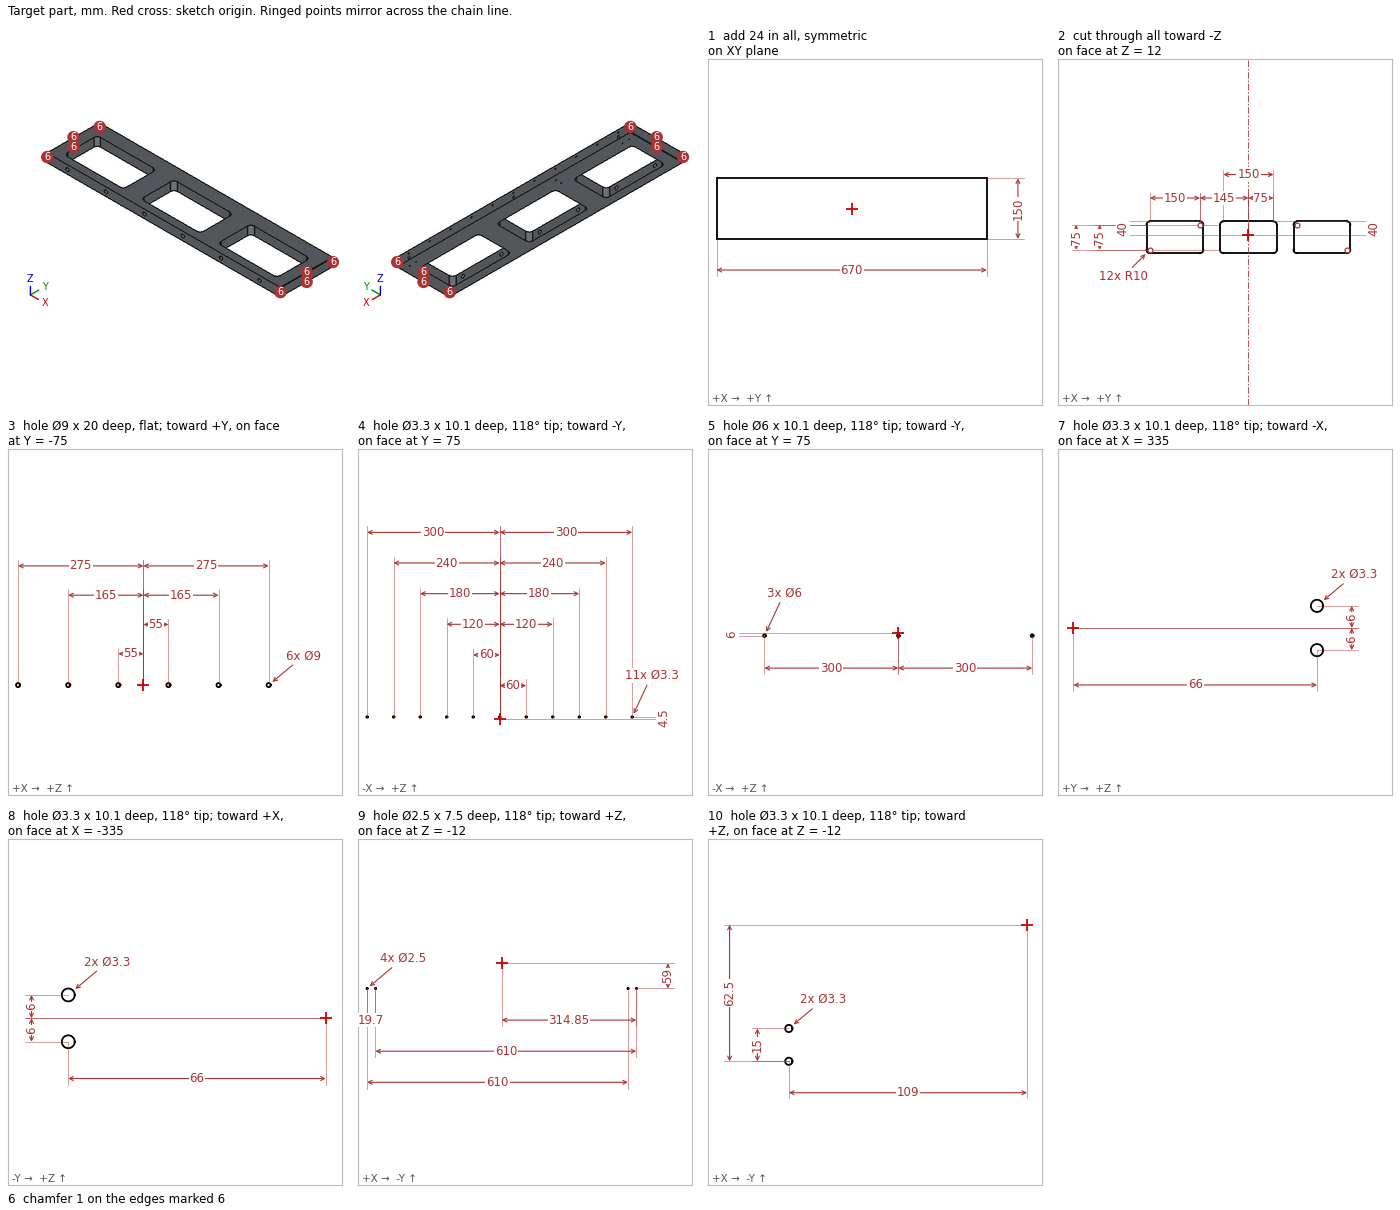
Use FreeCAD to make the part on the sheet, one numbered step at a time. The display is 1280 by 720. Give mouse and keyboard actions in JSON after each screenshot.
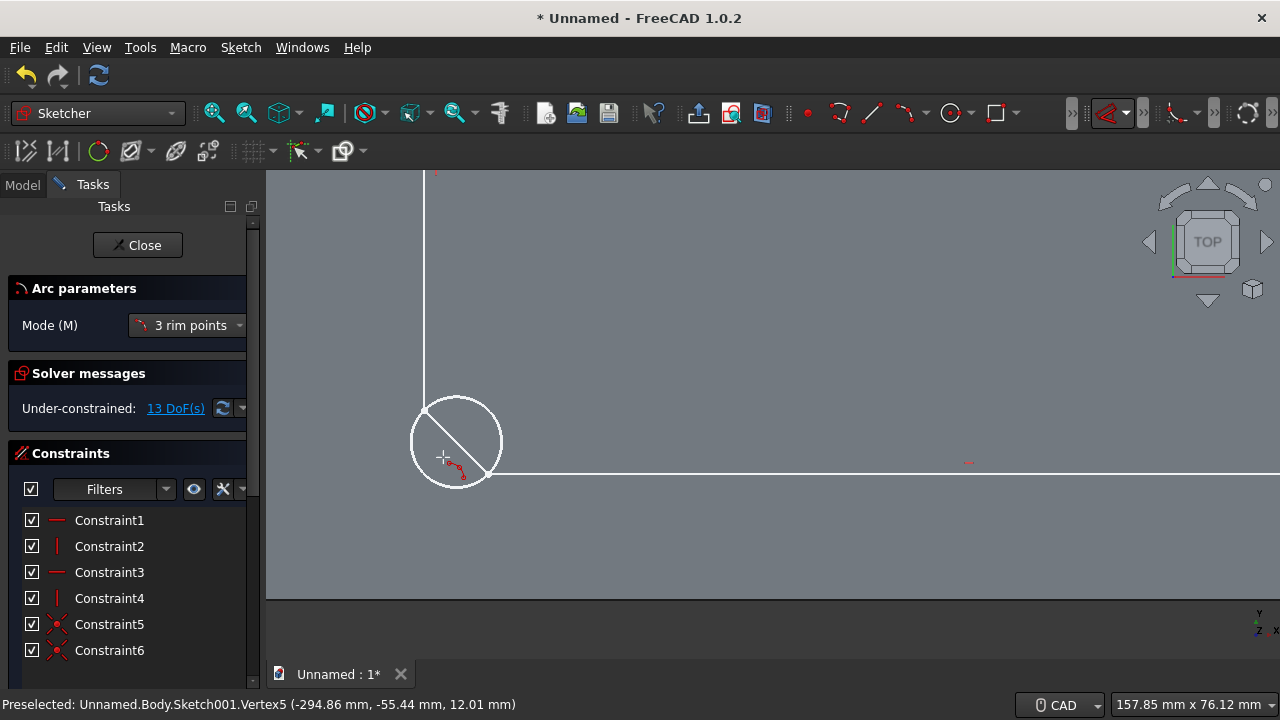
{"action": "left_click", "coordinate": [442, 453]}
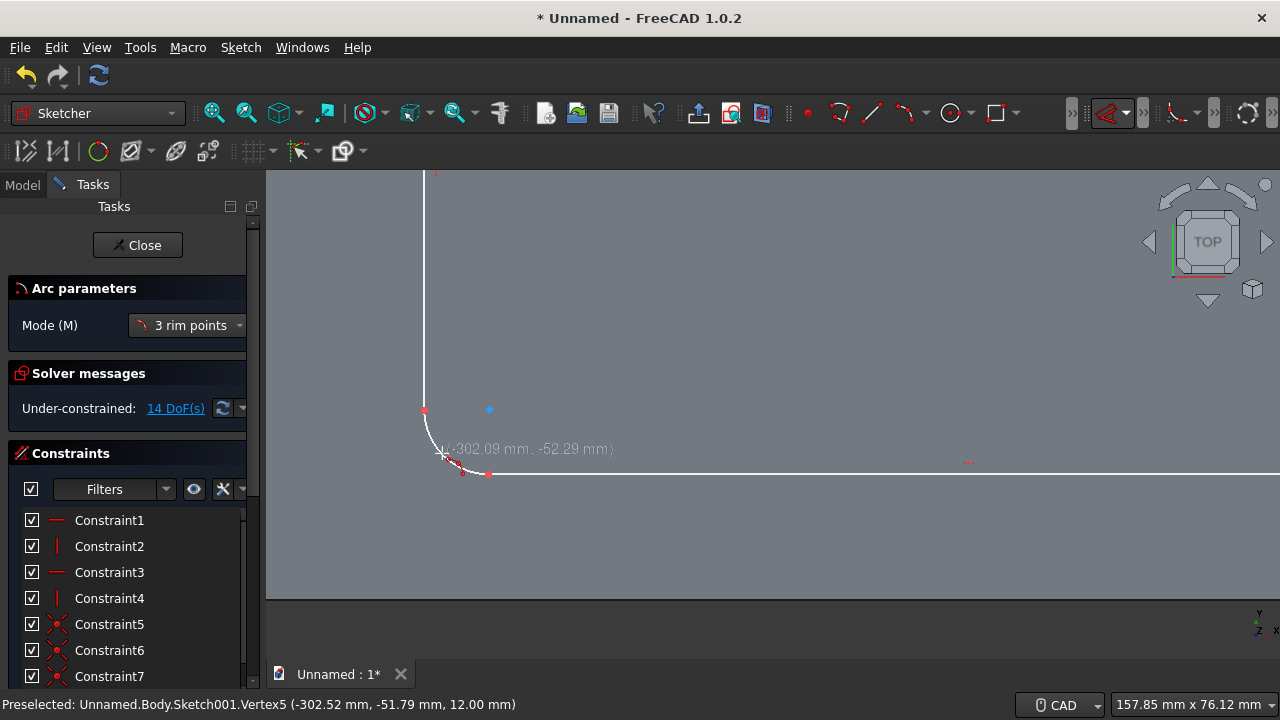
{"action": "scroll", "coordinate": [442, 453], "scroll_direction": "down", "scroll_amount": 10}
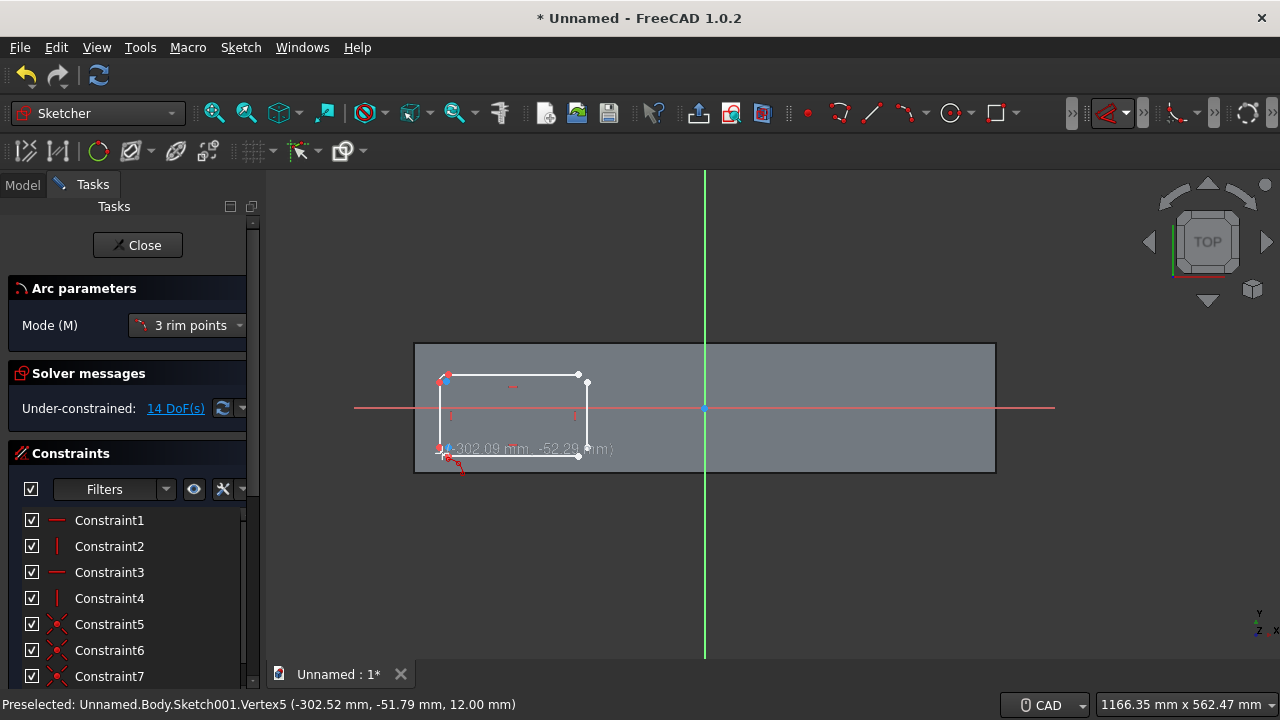
{"action": "scroll", "coordinate": [579, 456], "scroll_direction": "up", "scroll_amount": 2}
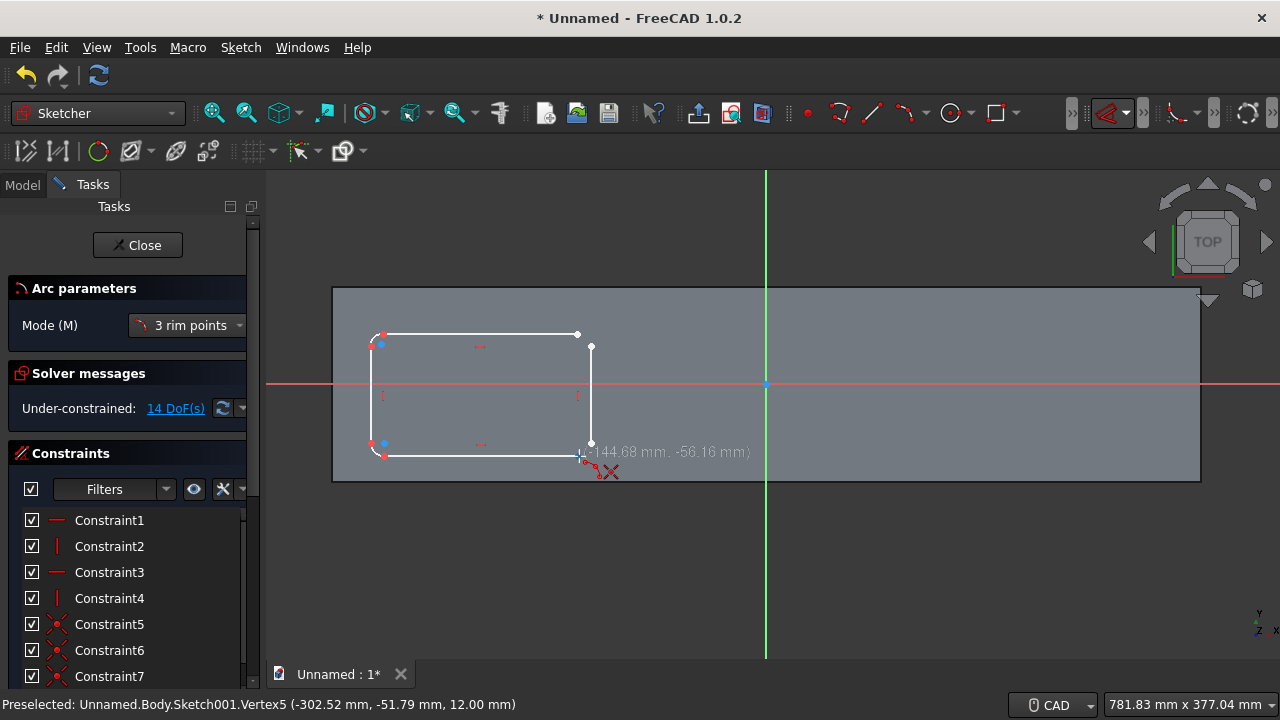
{"action": "left_click", "coordinate": [578, 456]}
{"action": "left_click", "coordinate": [591, 443]}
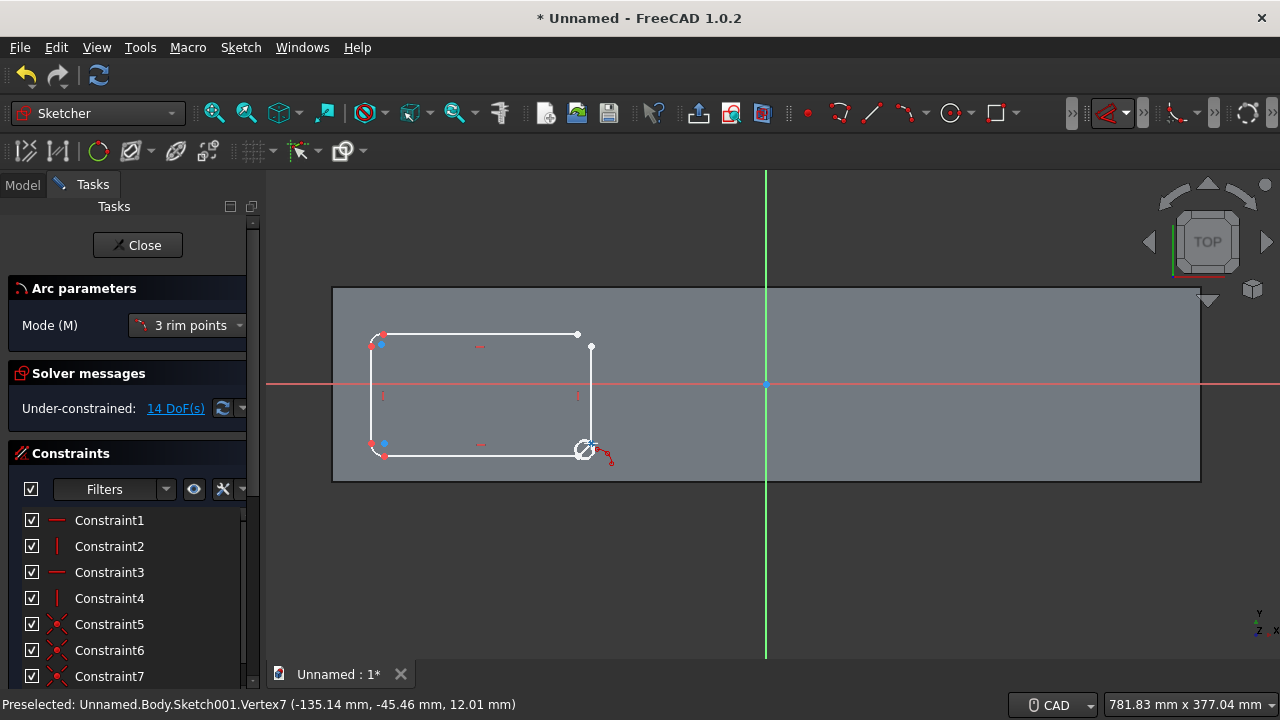
{"action": "scroll", "coordinate": [588, 452], "scroll_direction": "up", "scroll_amount": 8}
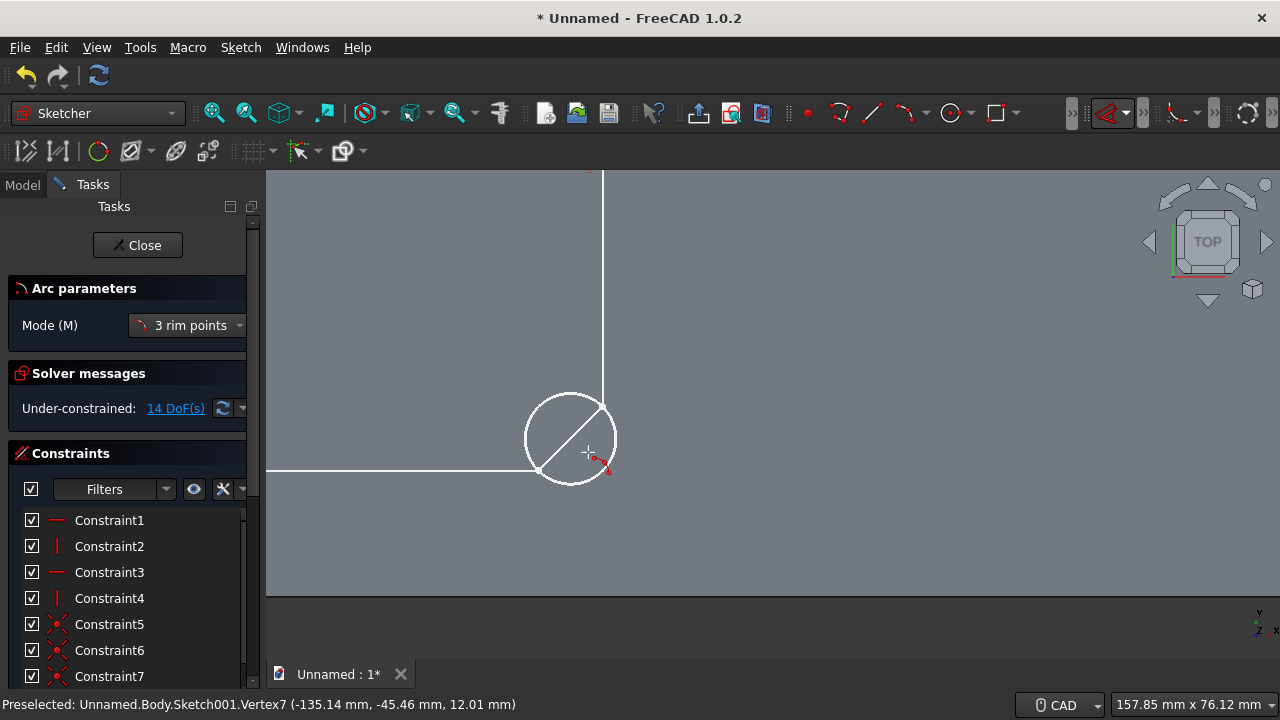
{"action": "left_click", "coordinate": [585, 449]}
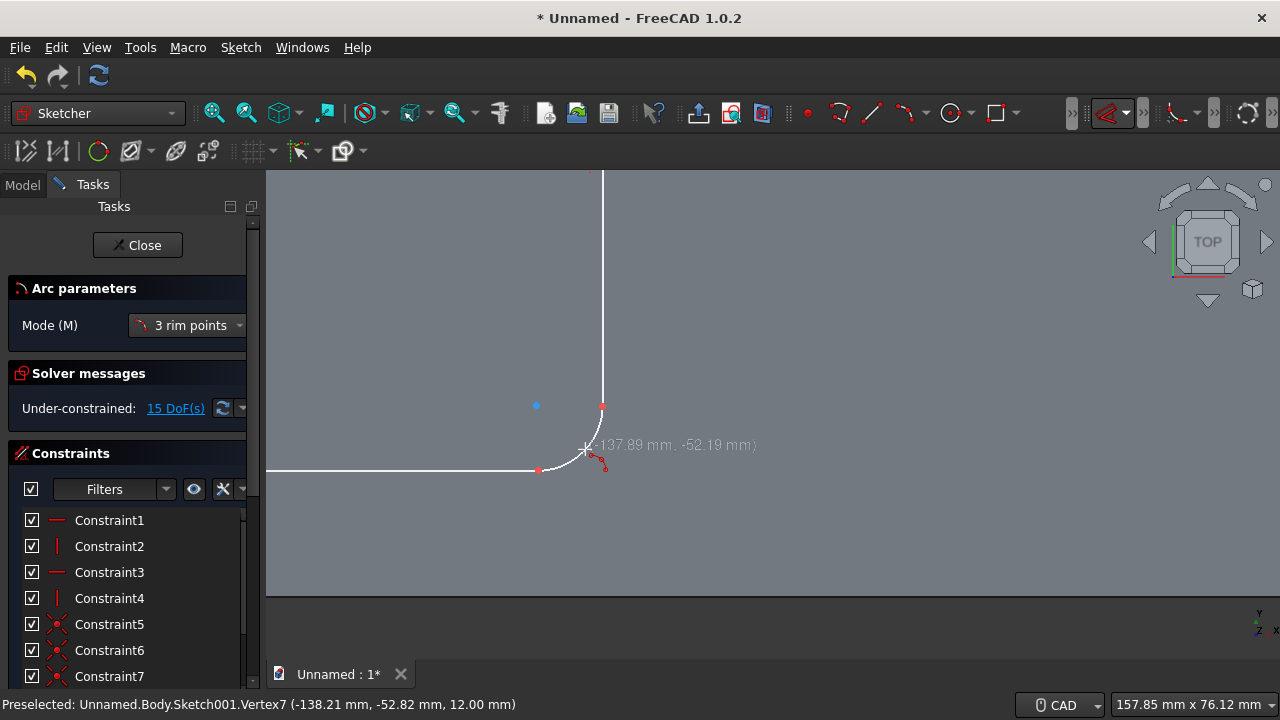
{"action": "scroll", "coordinate": [585, 454], "scroll_direction": "down", "scroll_amount": 10}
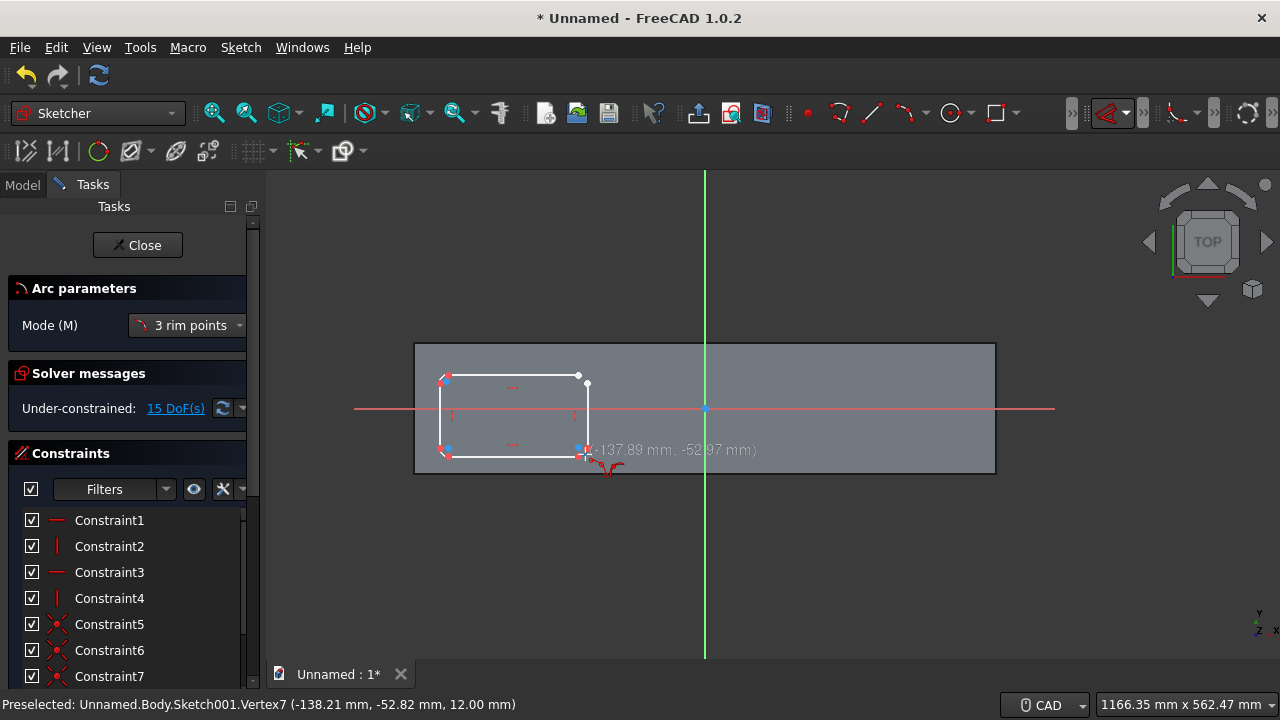
{"action": "scroll", "coordinate": [588, 383], "scroll_direction": "up", "scroll_amount": 2}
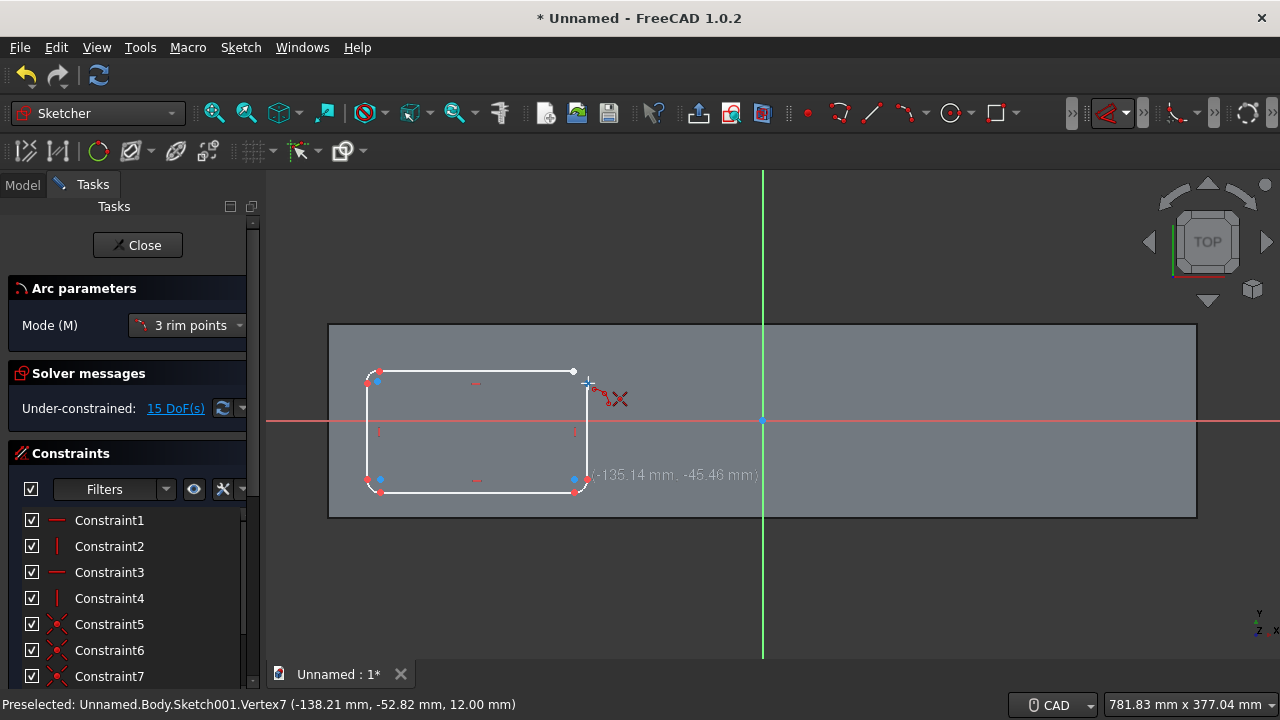
{"action": "left_click", "coordinate": [587, 383]}
{"action": "left_click", "coordinate": [574, 371]}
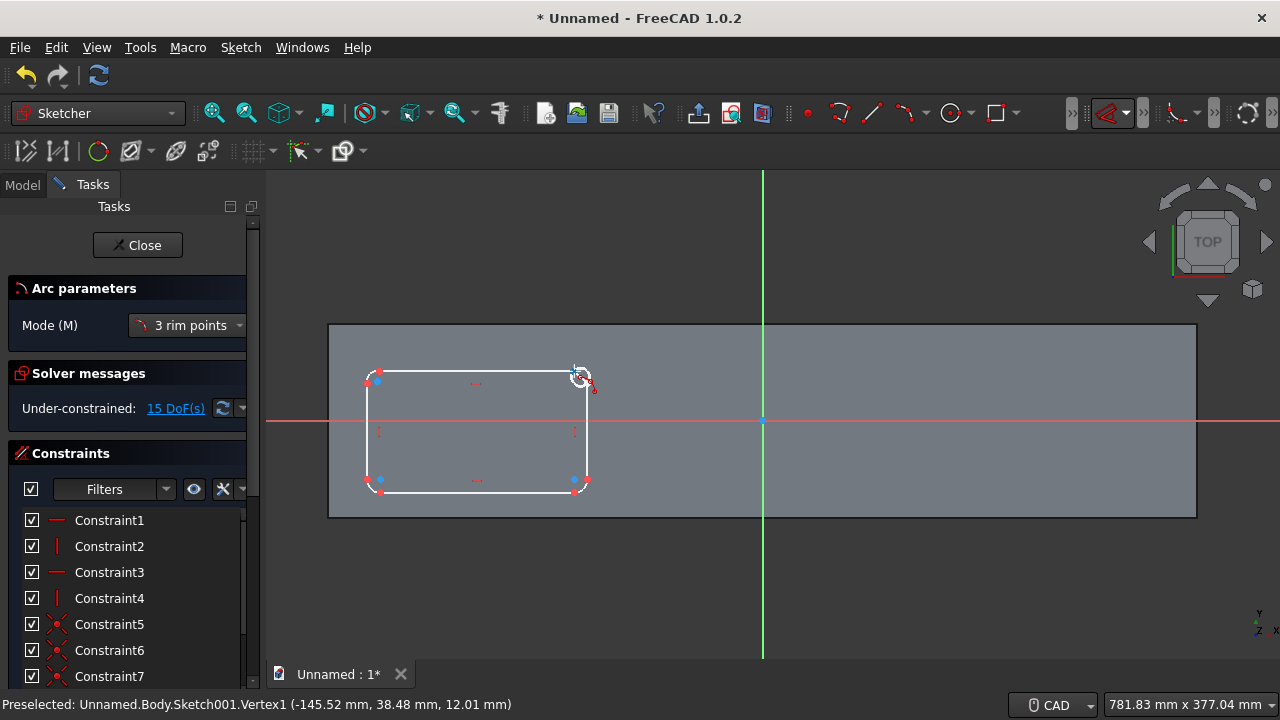
{"action": "scroll", "coordinate": [584, 373], "scroll_direction": "up", "scroll_amount": 8}